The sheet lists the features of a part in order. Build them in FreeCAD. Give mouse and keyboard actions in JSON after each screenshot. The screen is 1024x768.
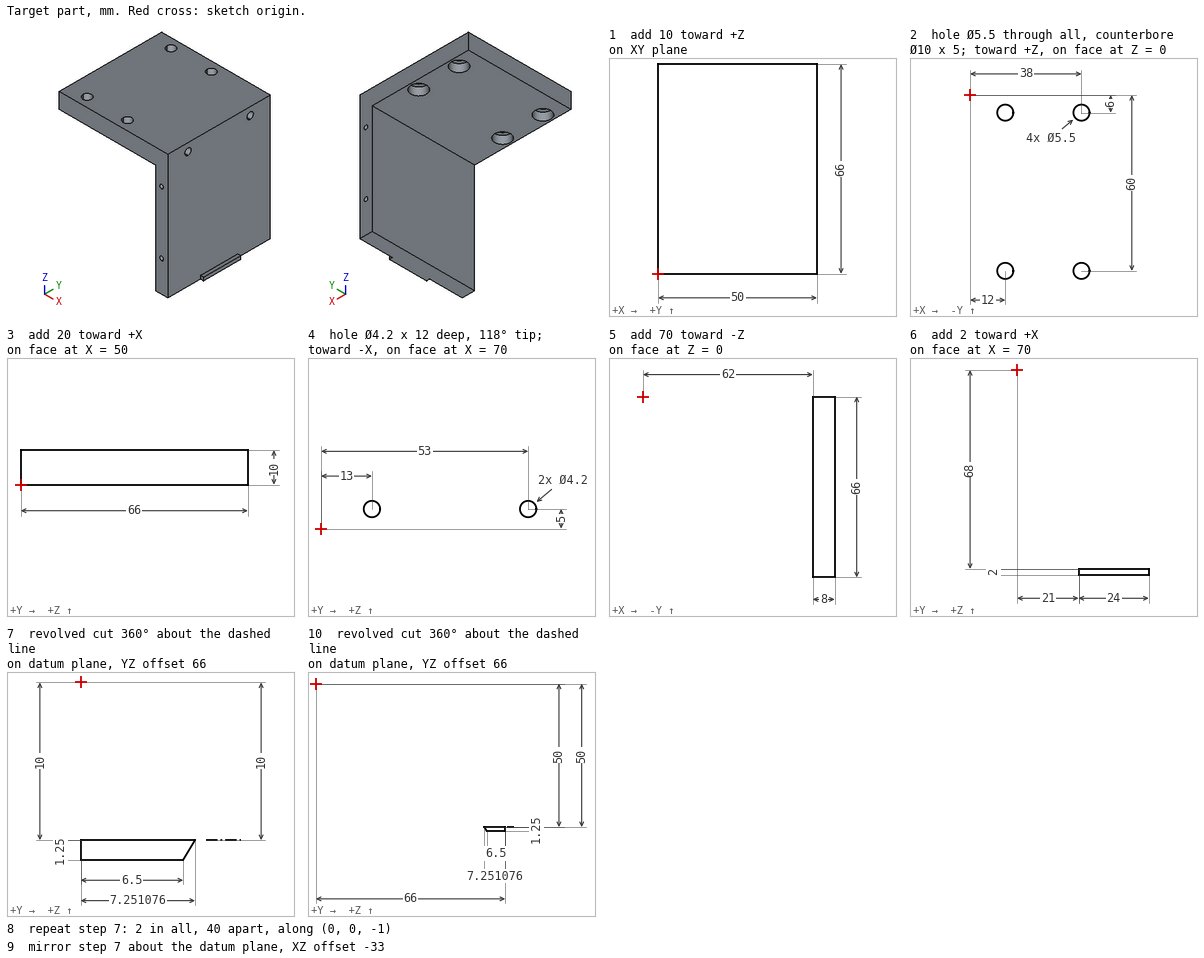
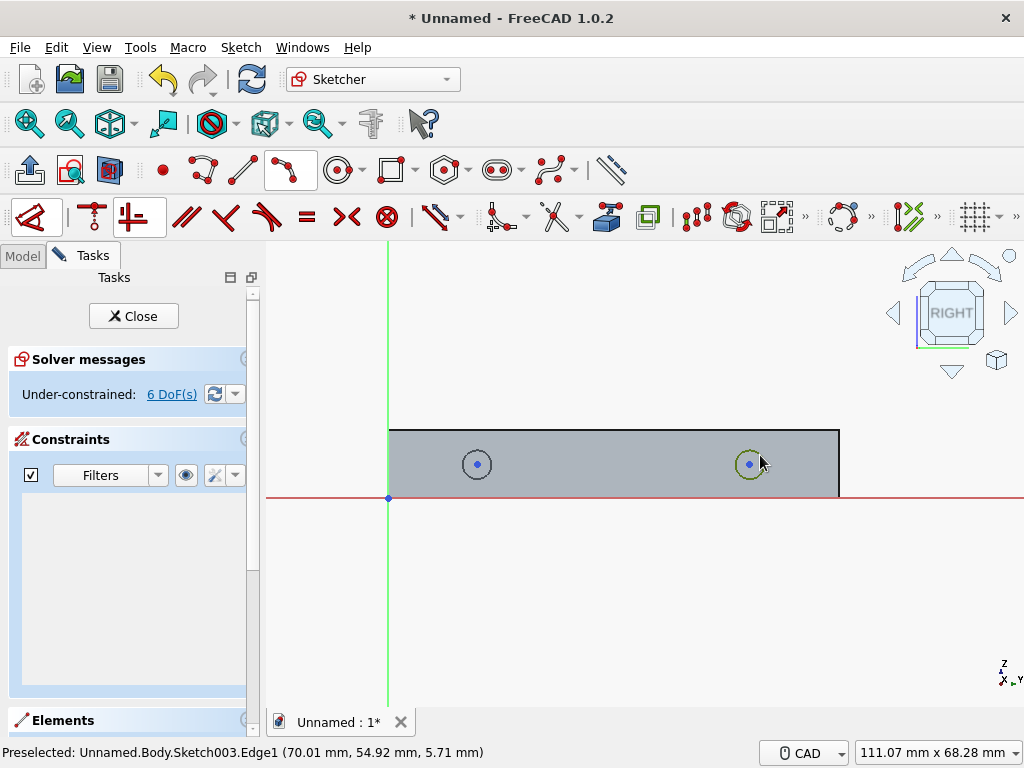
{"action": "left_click", "coordinate": [487, 455]}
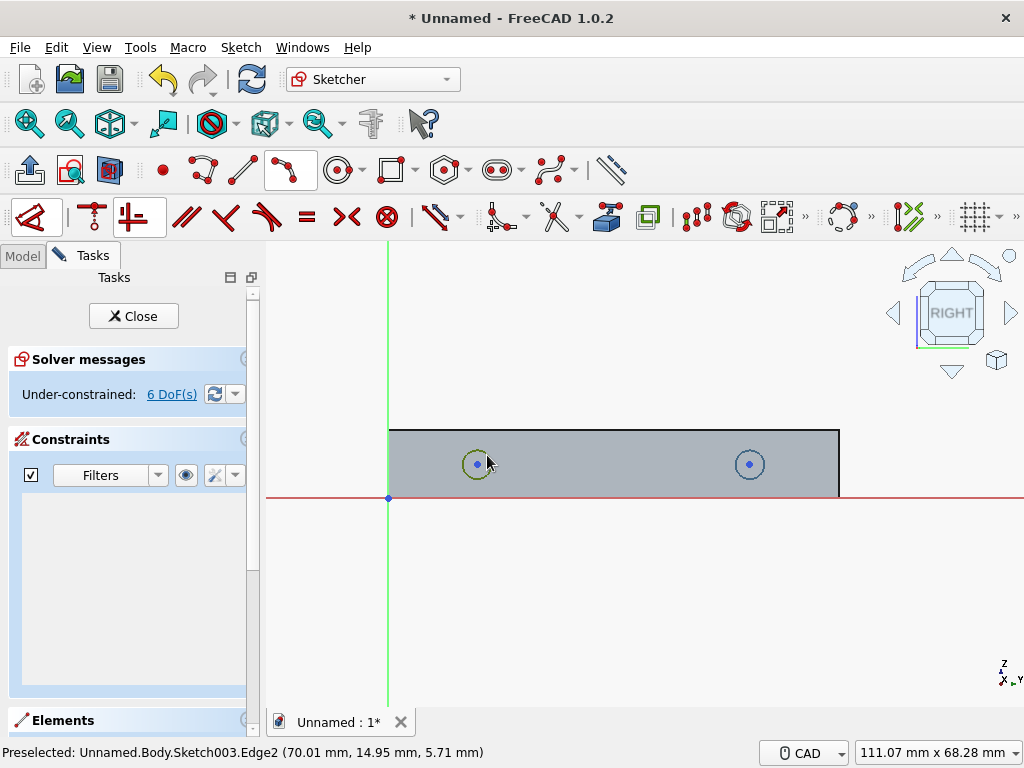
{"action": "key", "text": "e"}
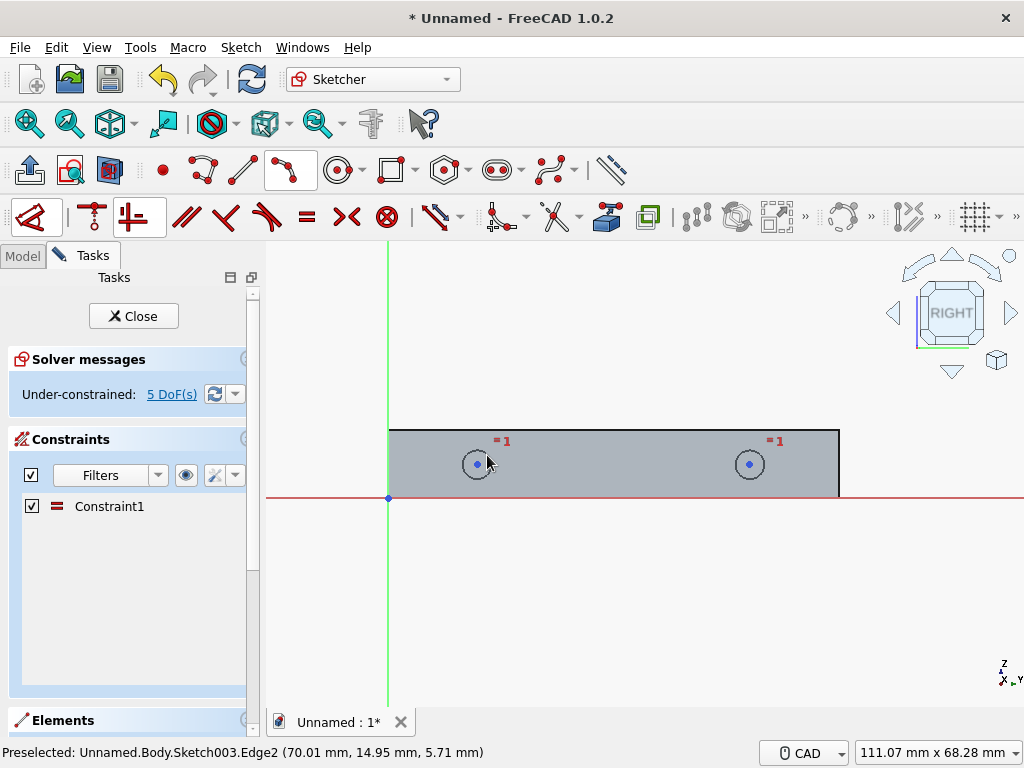
{"action": "left_click", "coordinate": [750, 465]}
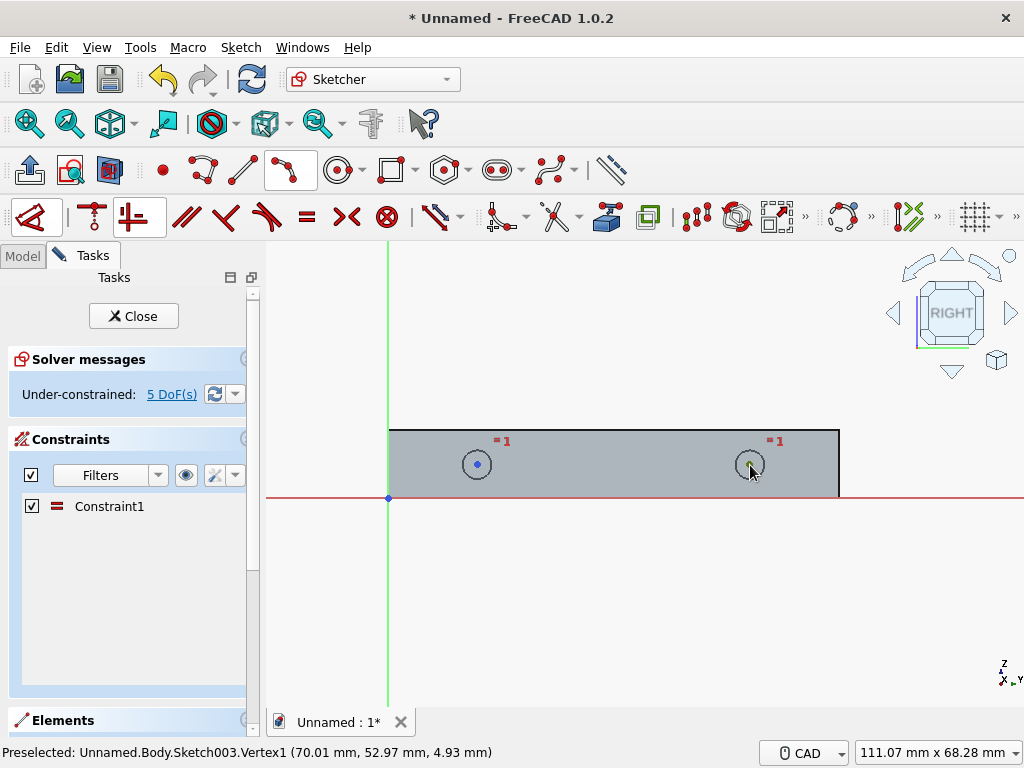
{"action": "left_click", "coordinate": [477, 465]}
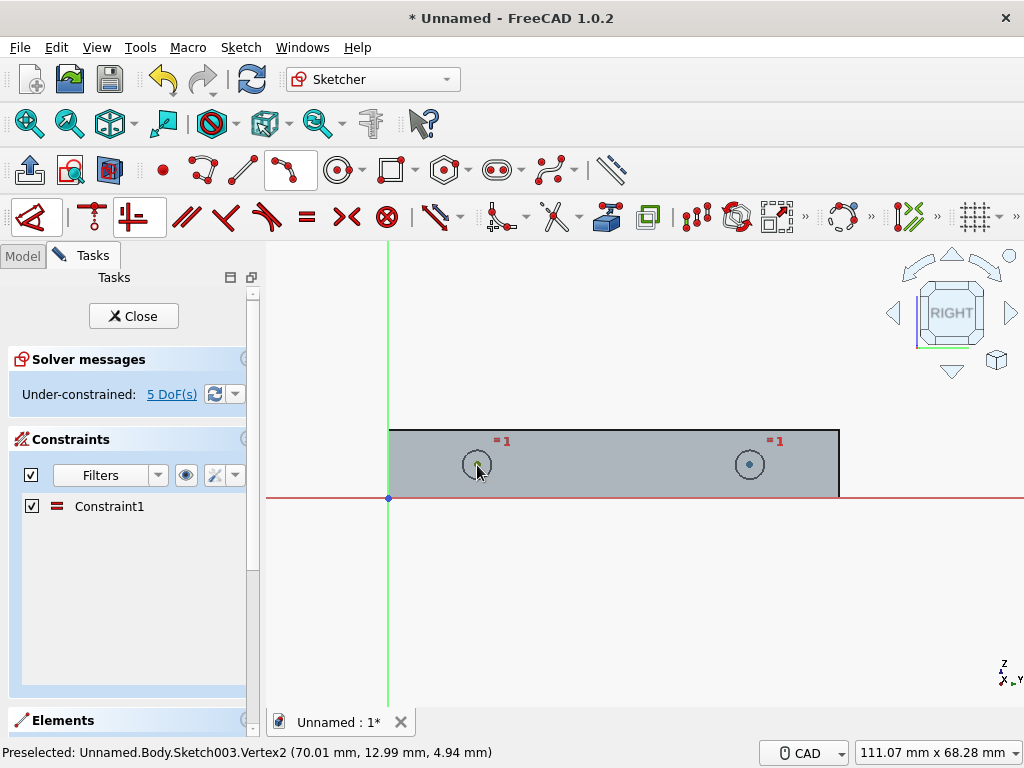
{"action": "key", "text": "h"}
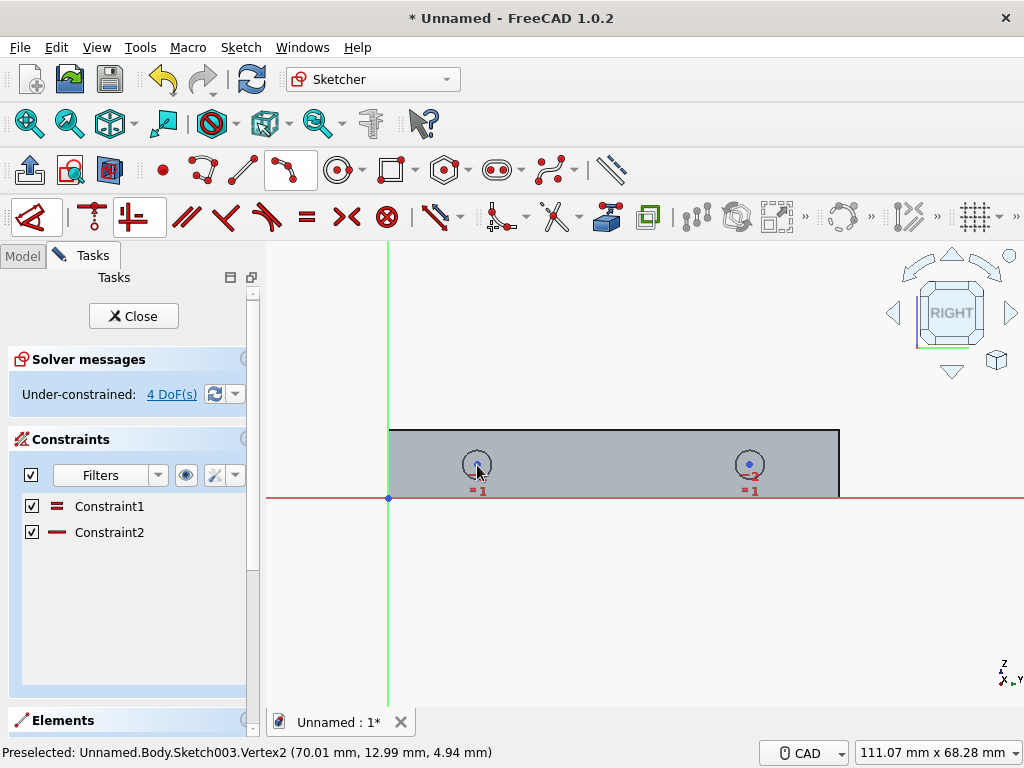
{"action": "scroll", "coordinate": [760, 455], "scroll_direction": "up", "scroll_amount": 2}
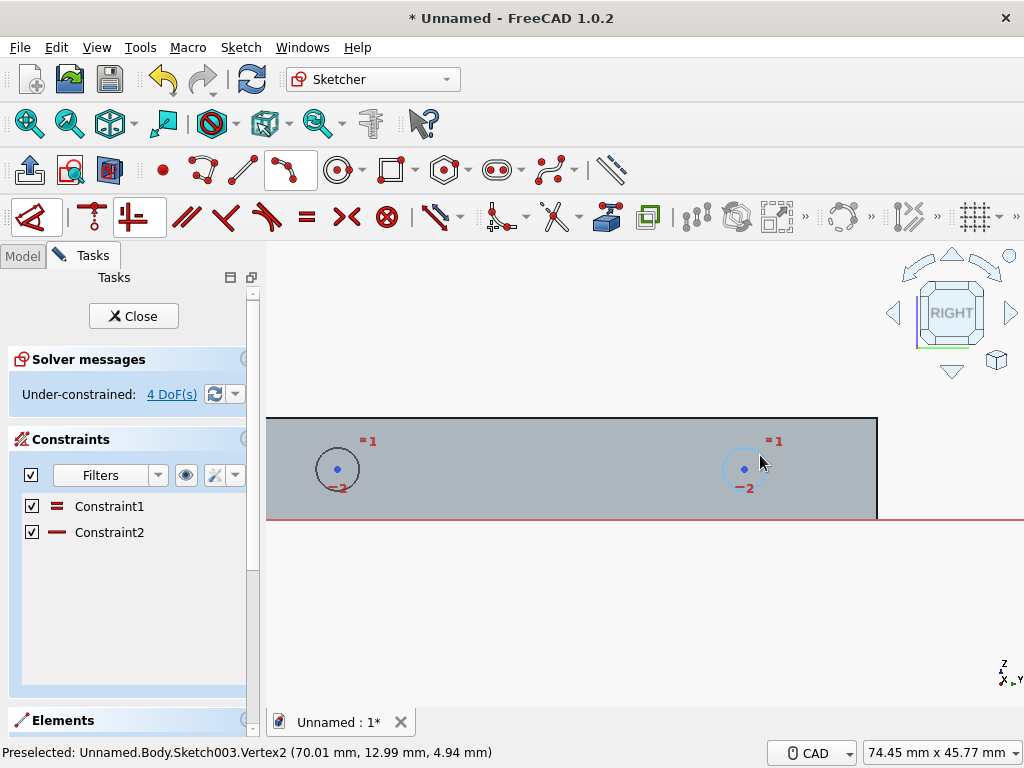
{"action": "left_click", "coordinate": [760, 454]}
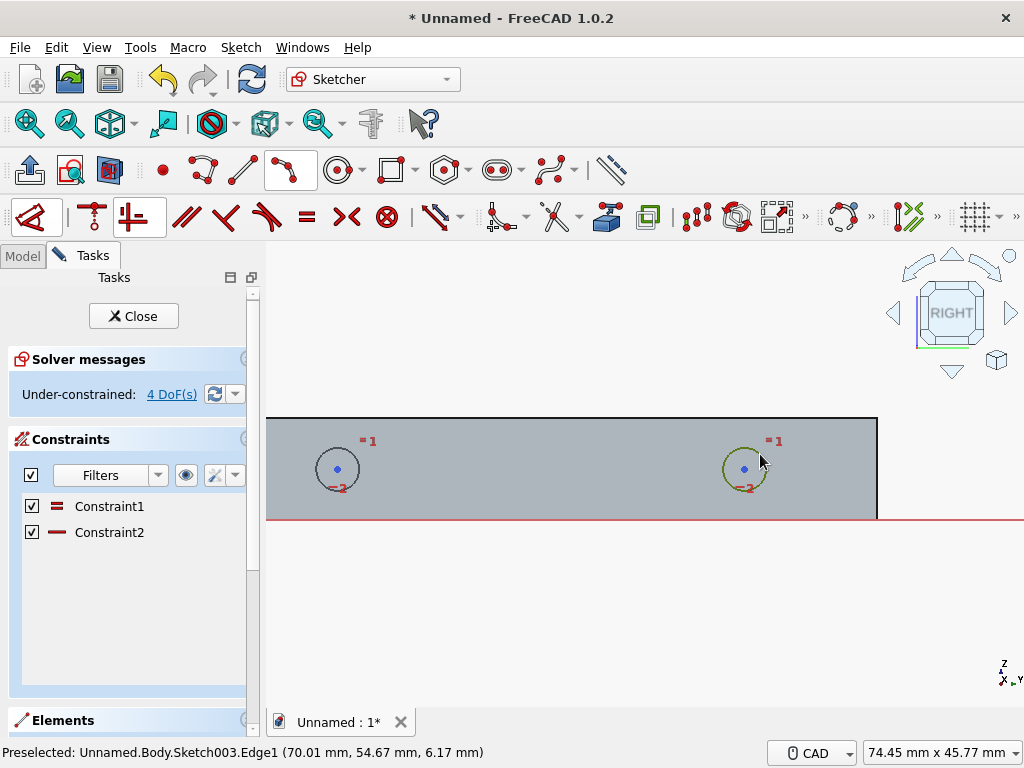
{"action": "key", "text": "k o"}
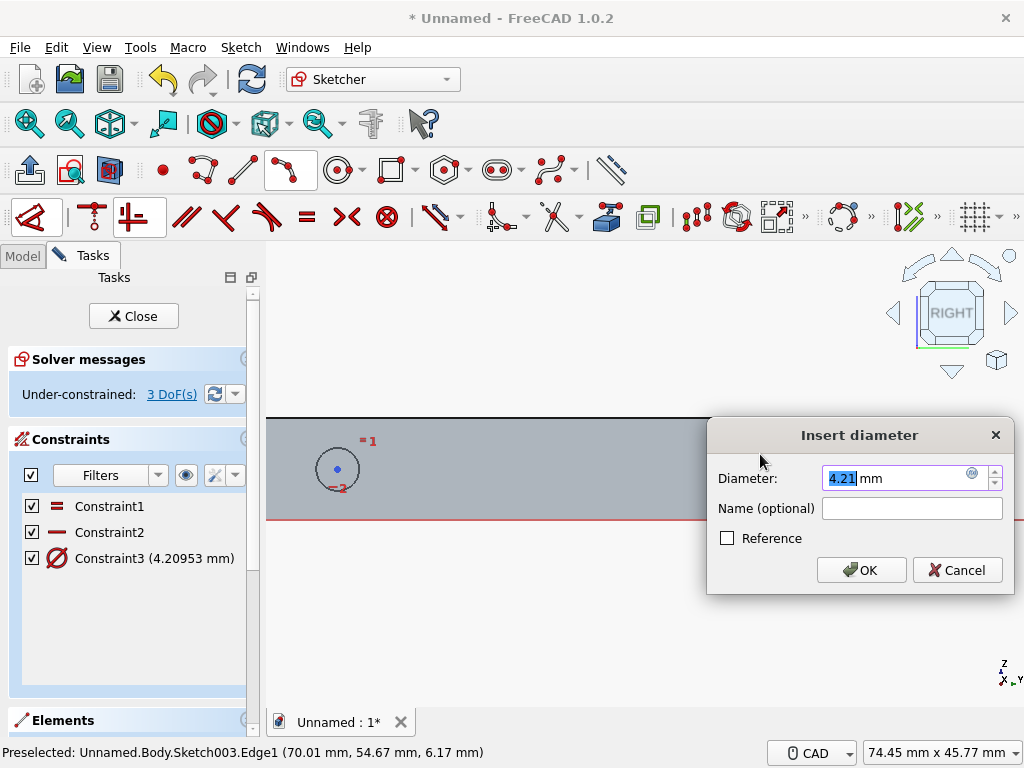
{"action": "type", "text": "4.2"}
{"action": "key", "text": "Return"}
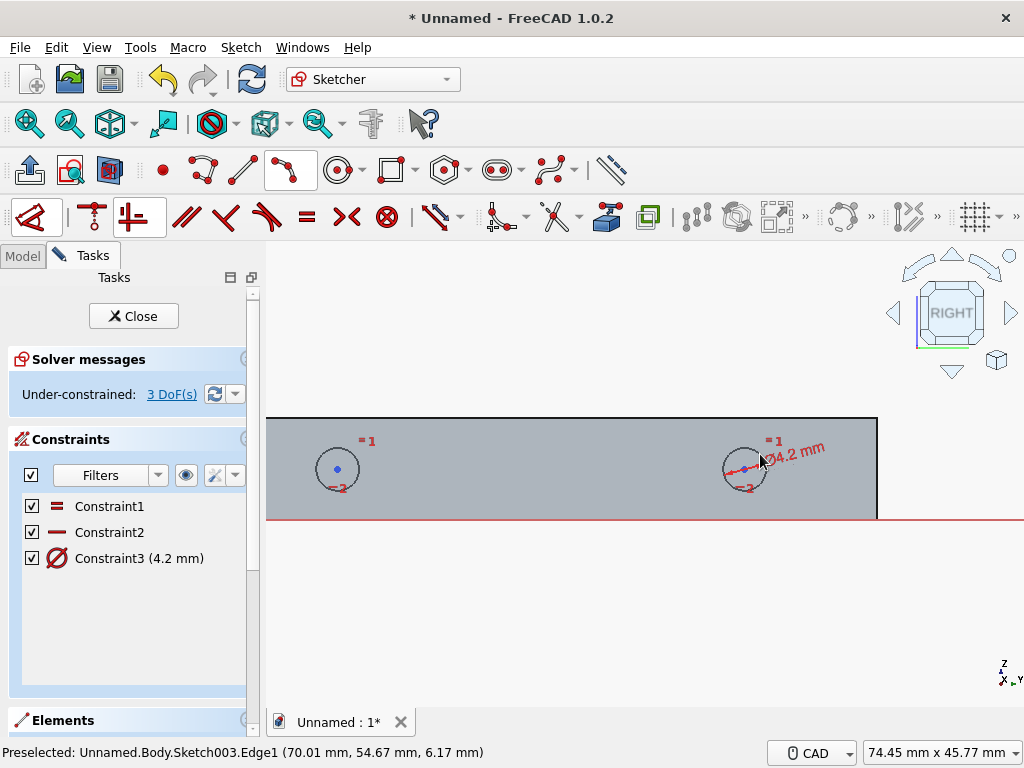
{"action": "left_click", "coordinate": [745, 469]}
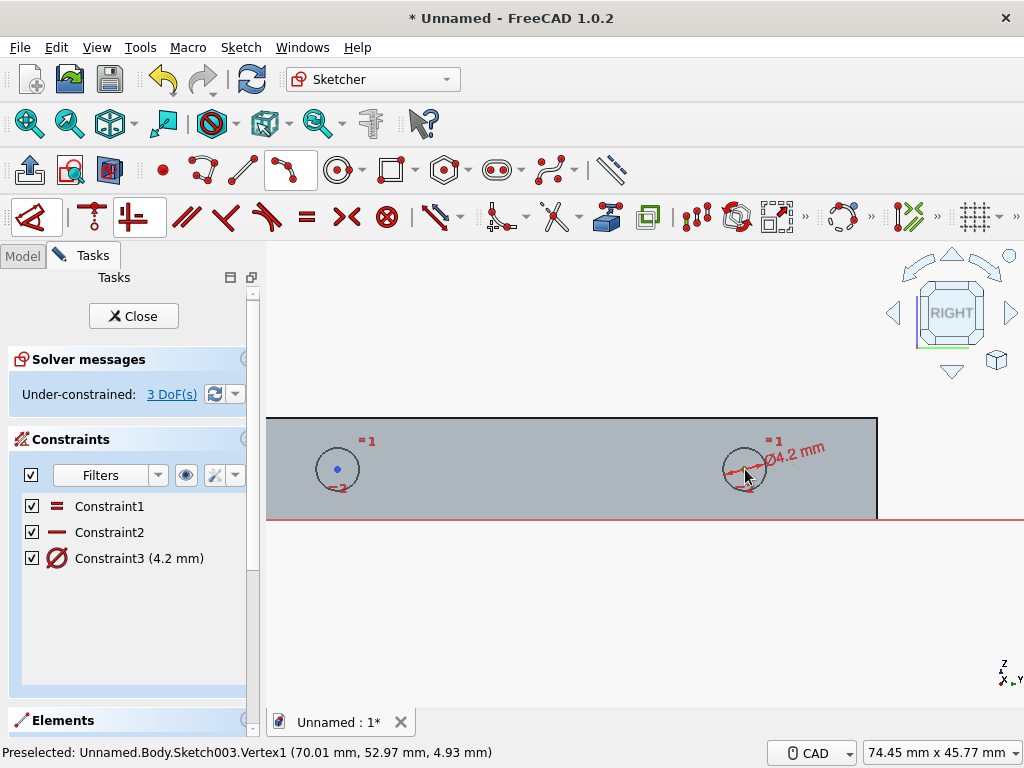
{"action": "key", "text": "i"}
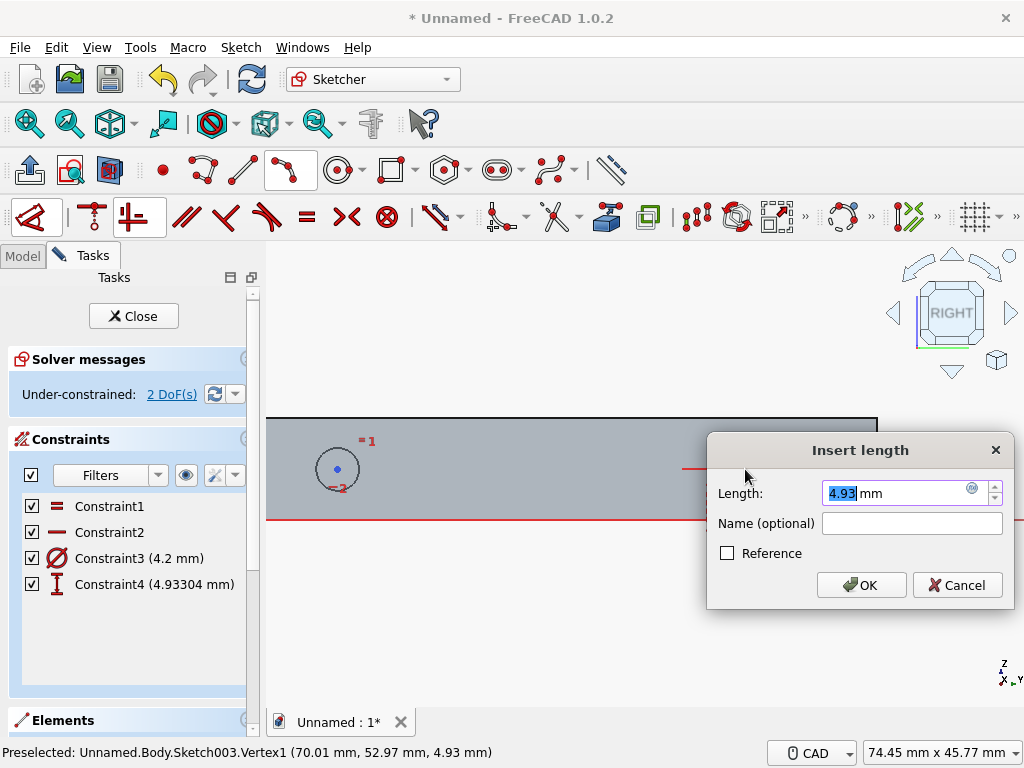
{"action": "type", "text": "5"}
{"action": "key", "text": "Return"}